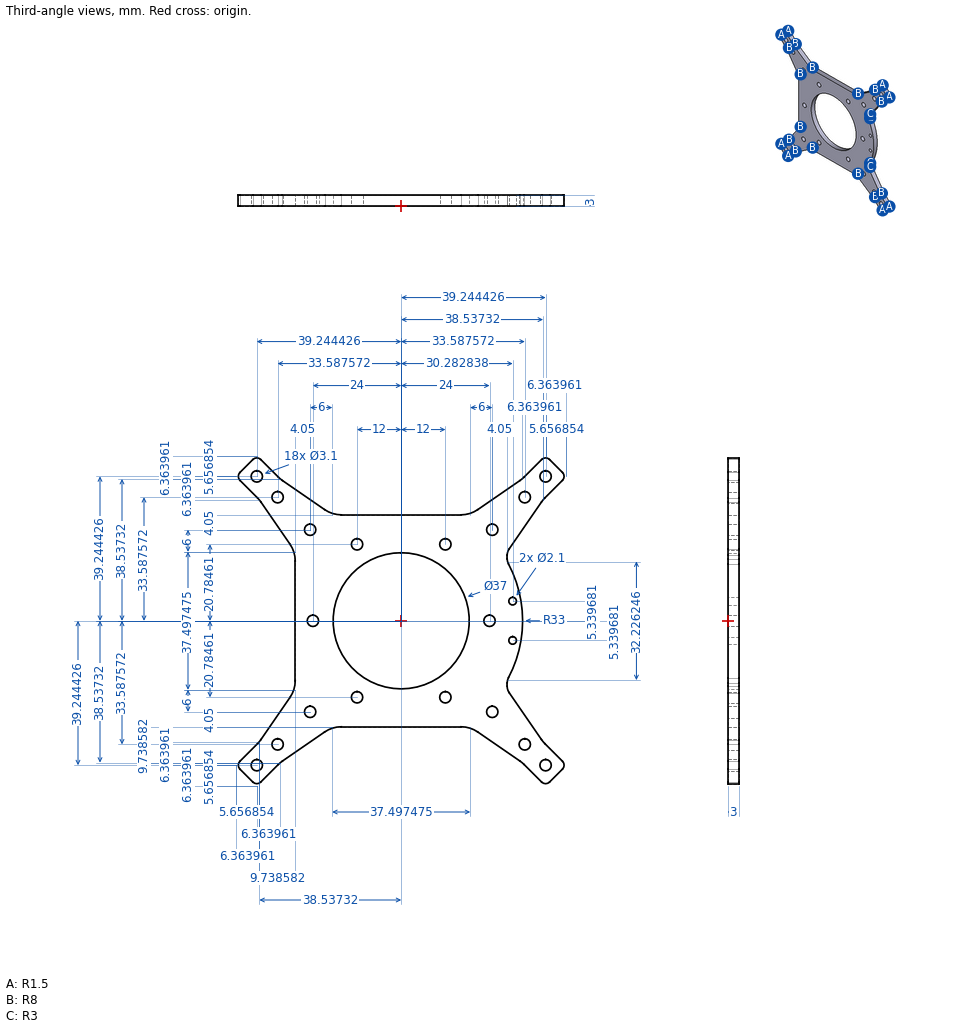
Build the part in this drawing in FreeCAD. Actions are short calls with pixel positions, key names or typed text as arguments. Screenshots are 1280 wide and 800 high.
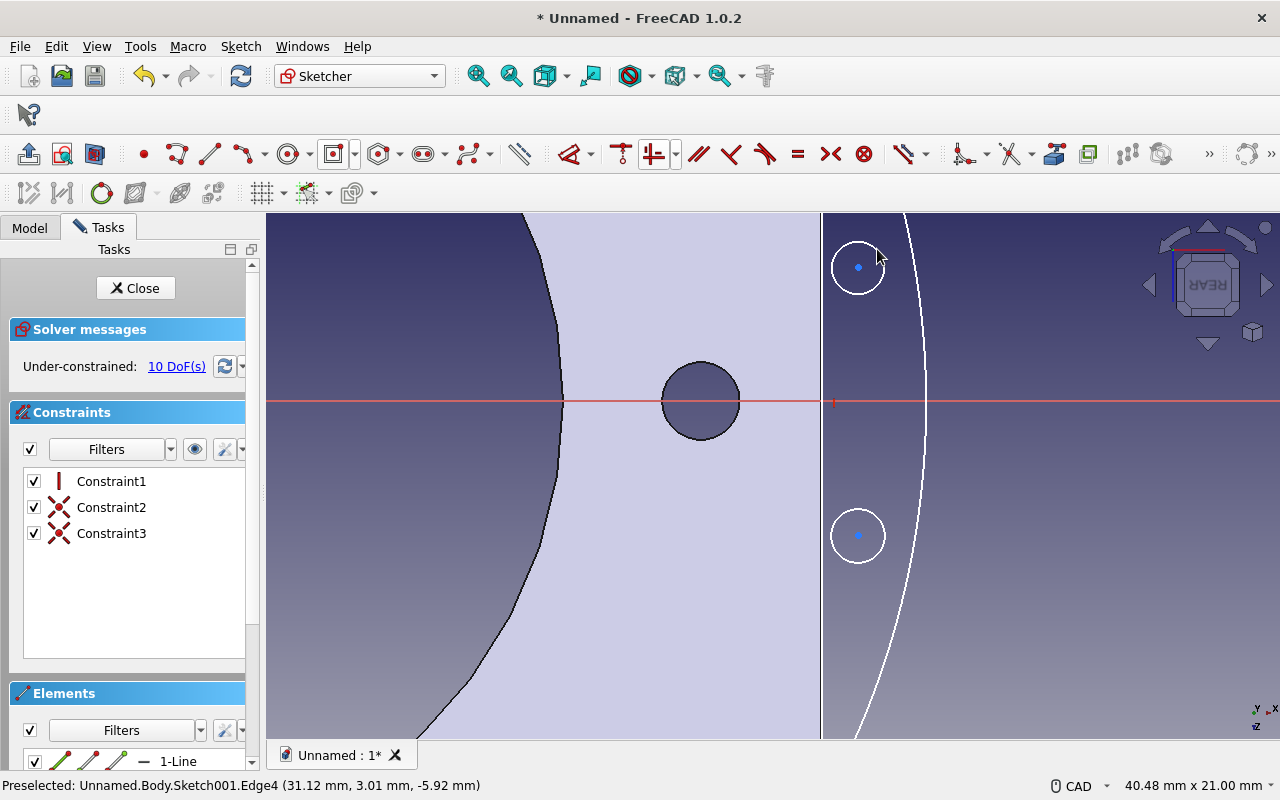
scroll(861, 537, down, 4)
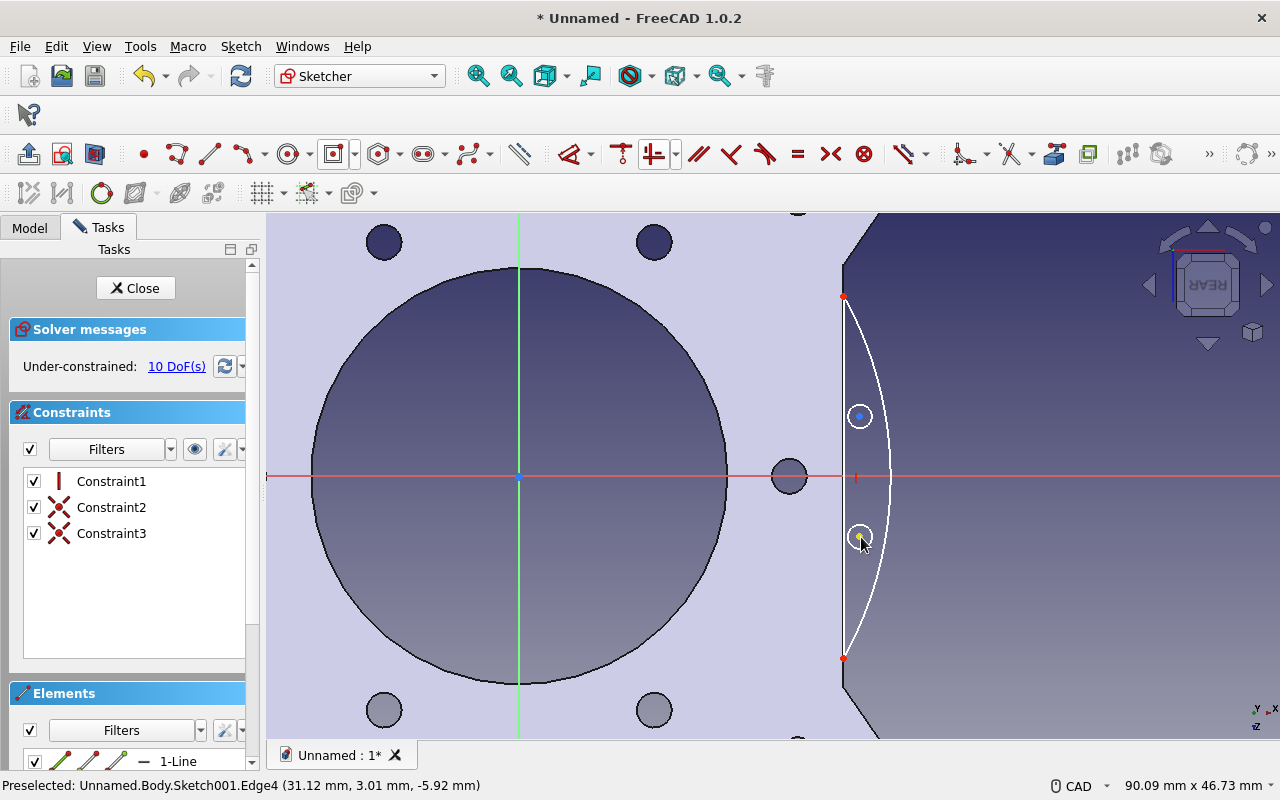
scroll(519, 477, up, 7)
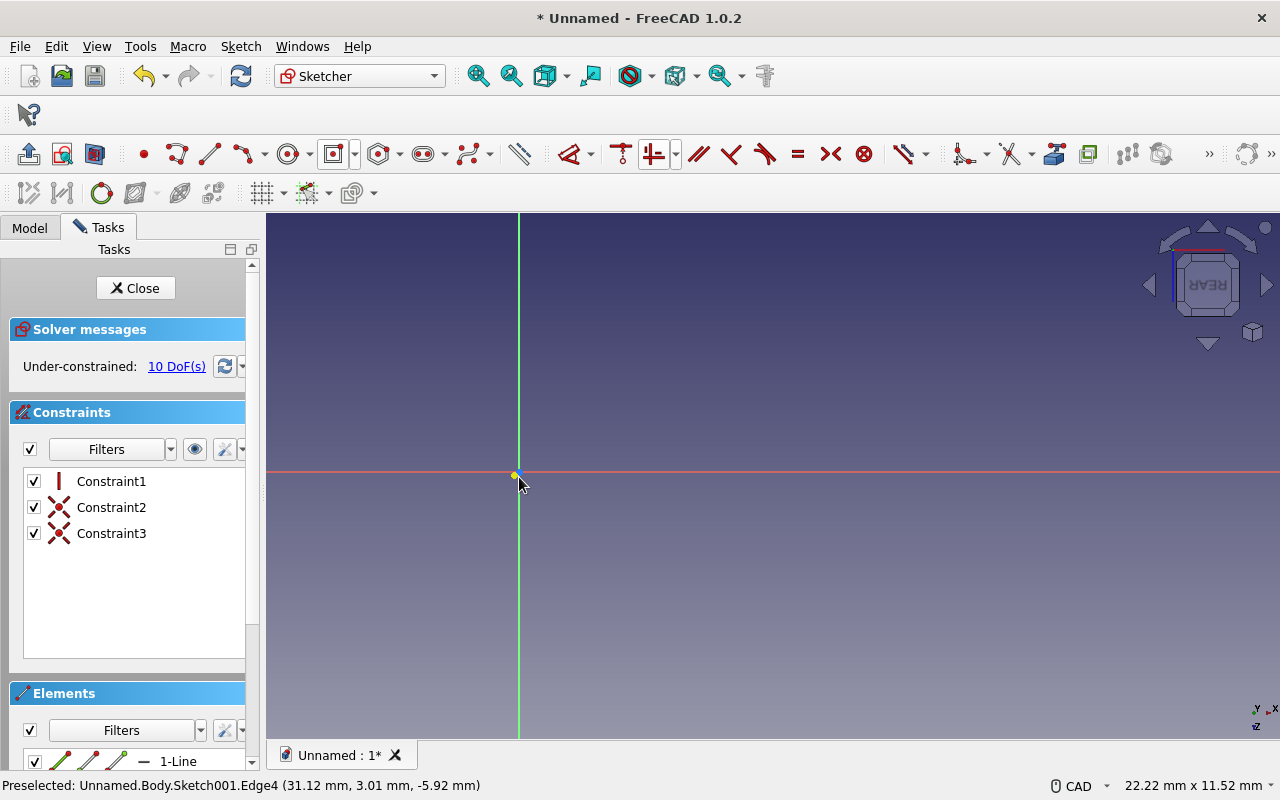
drag(505, 462, 529, 486)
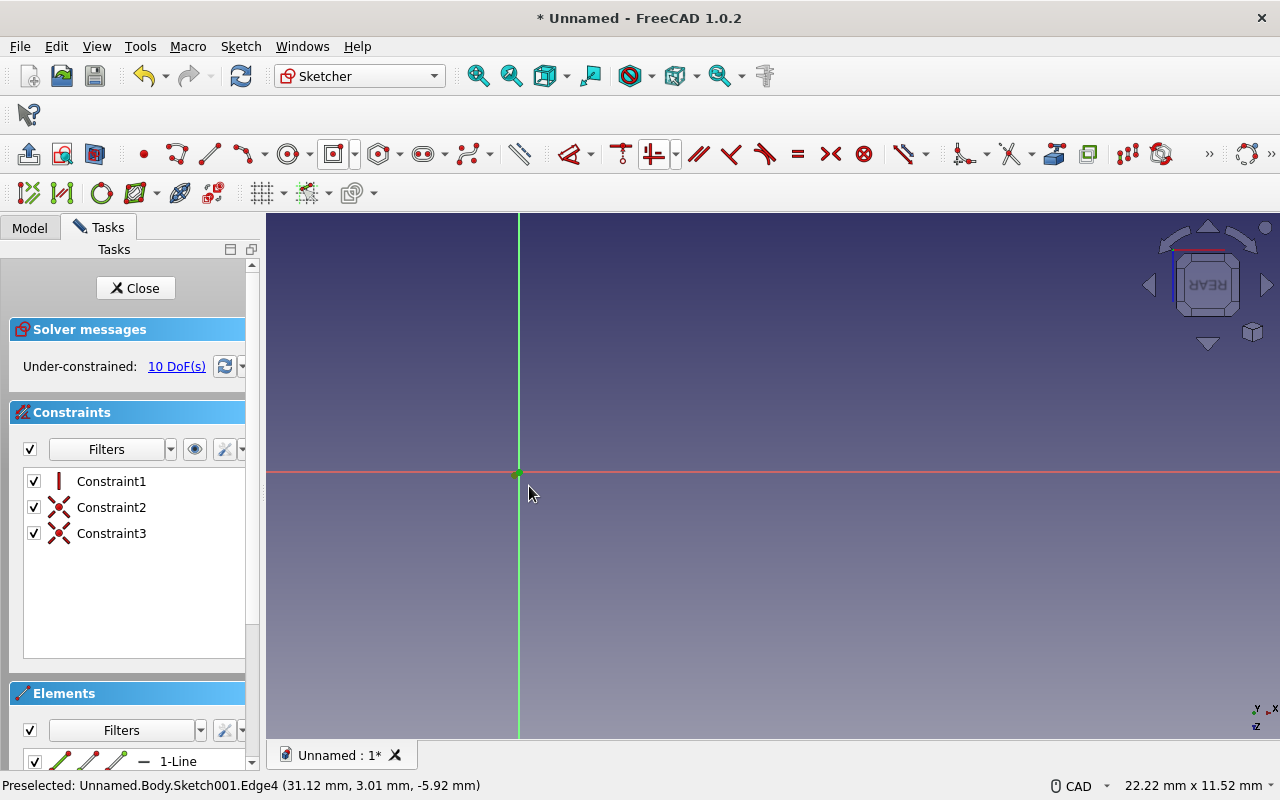
click(621, 154)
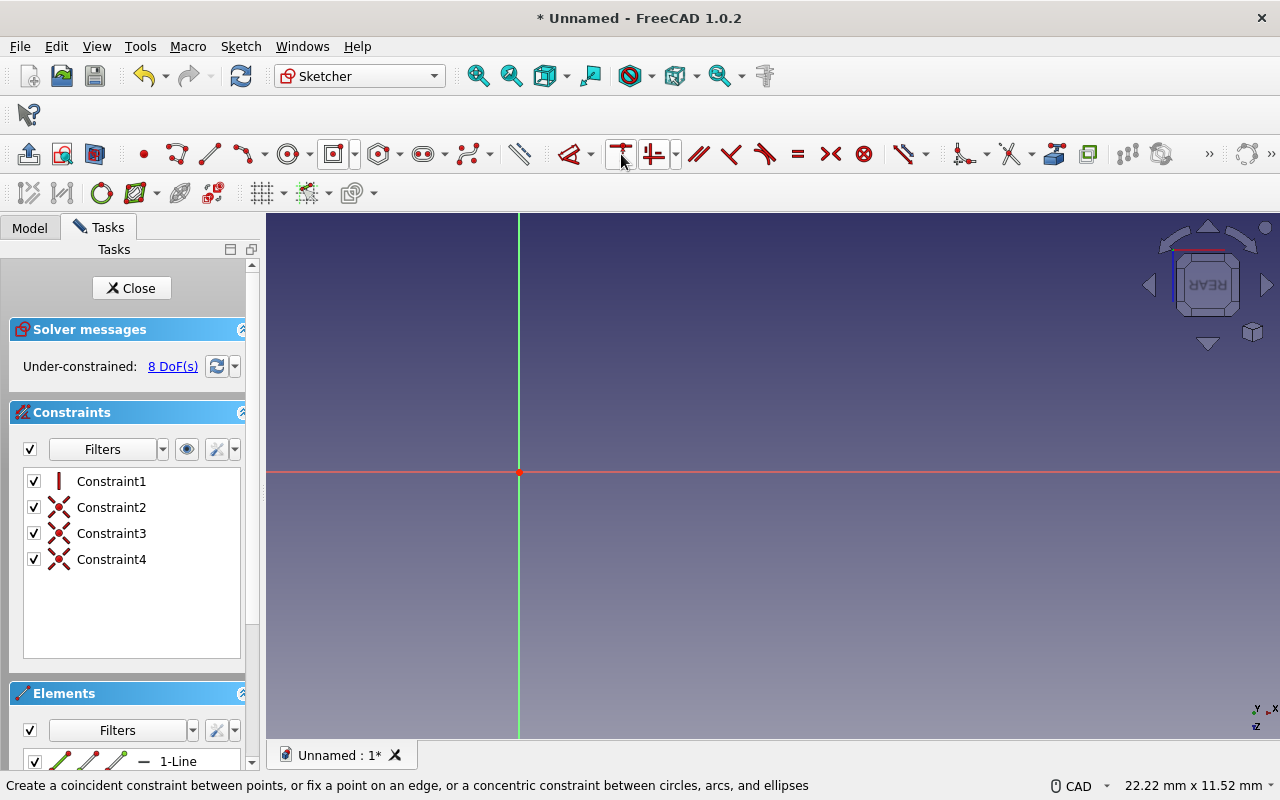
scroll(519, 477, down, 7)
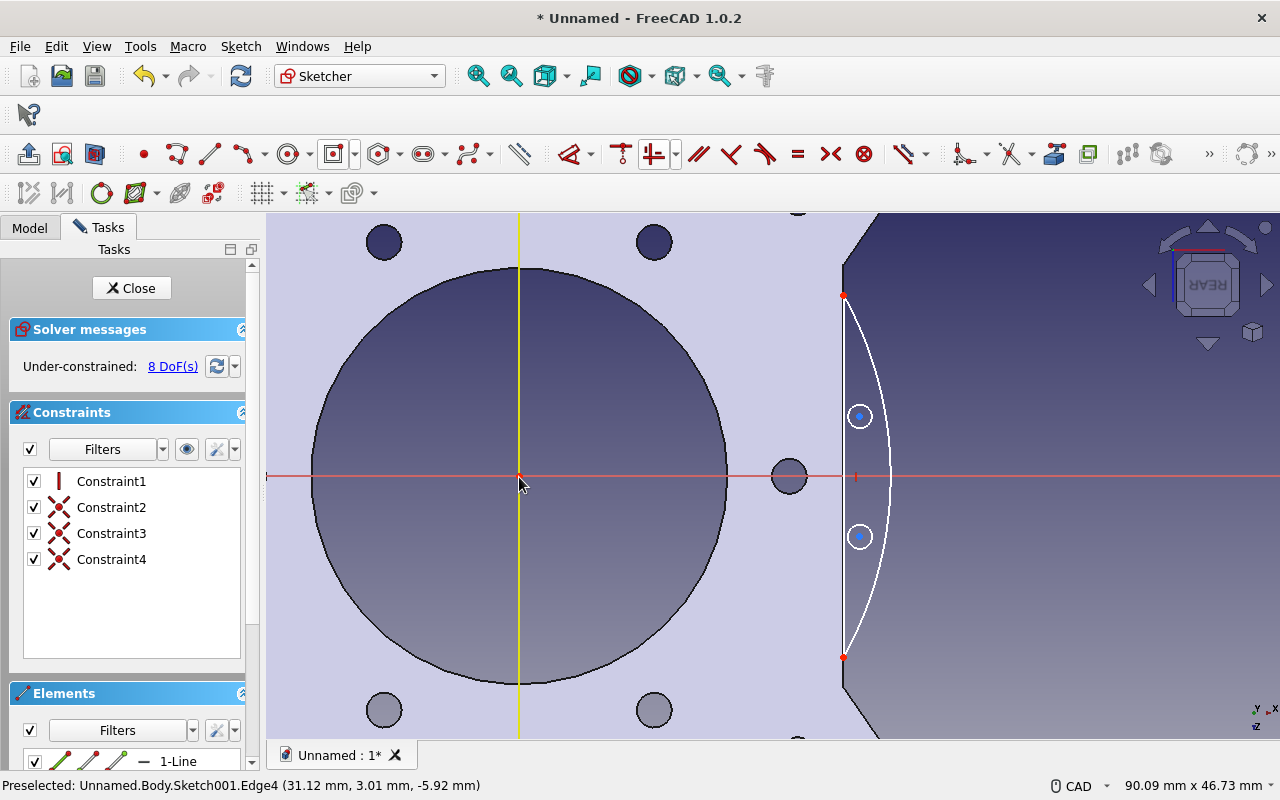
click(868, 528)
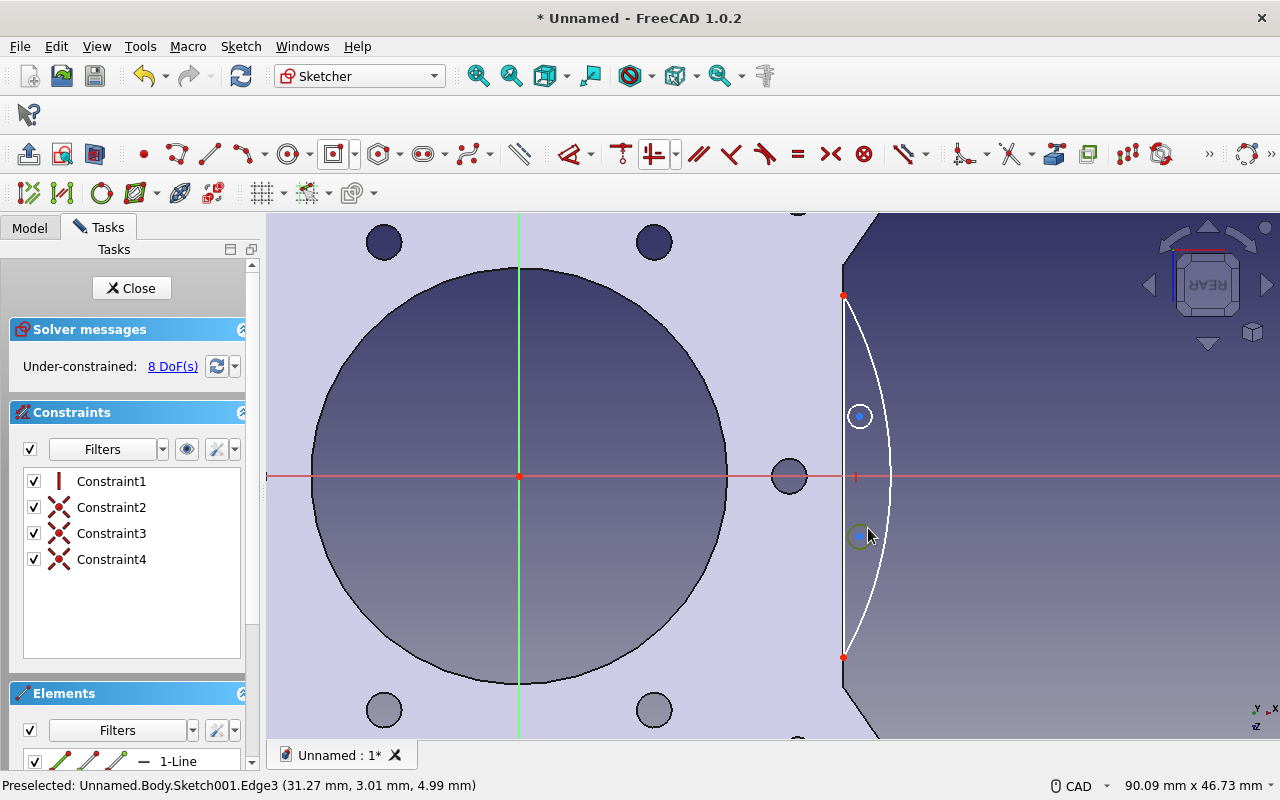
click(868, 408)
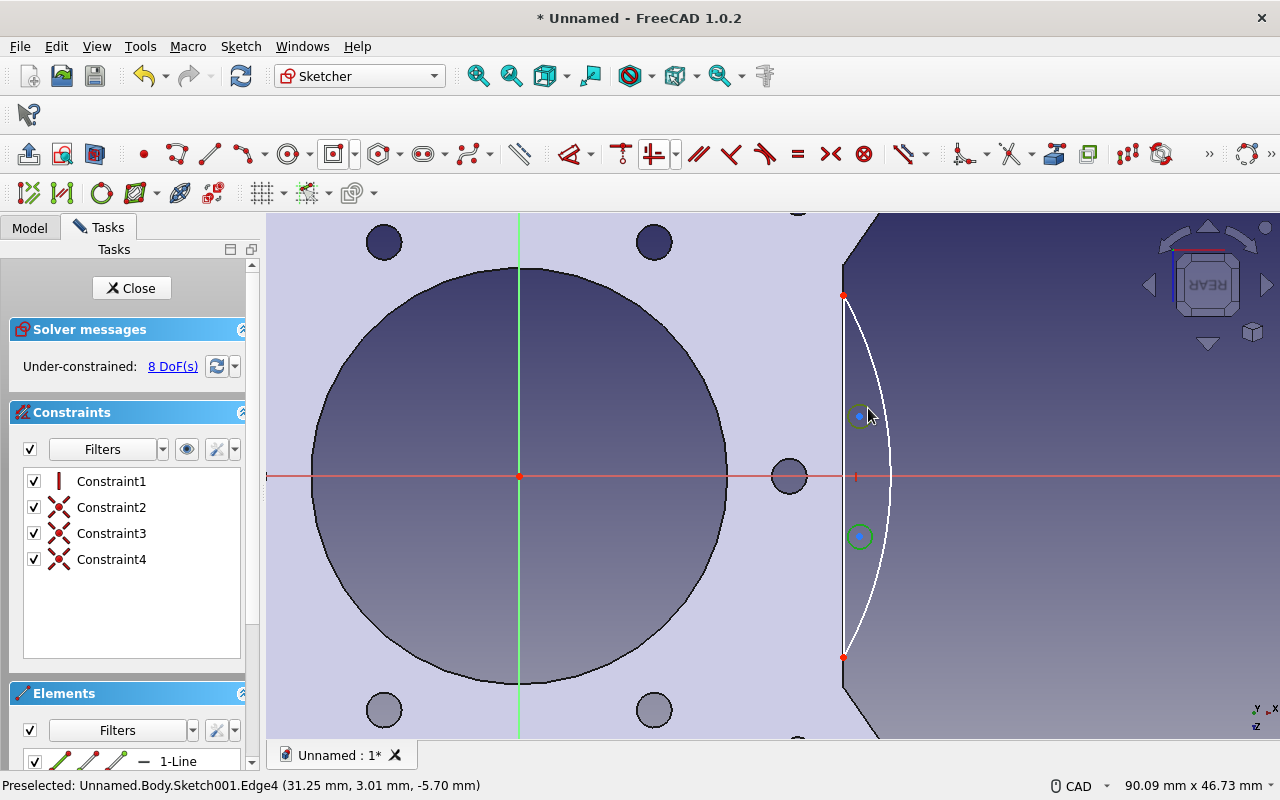
click(798, 154)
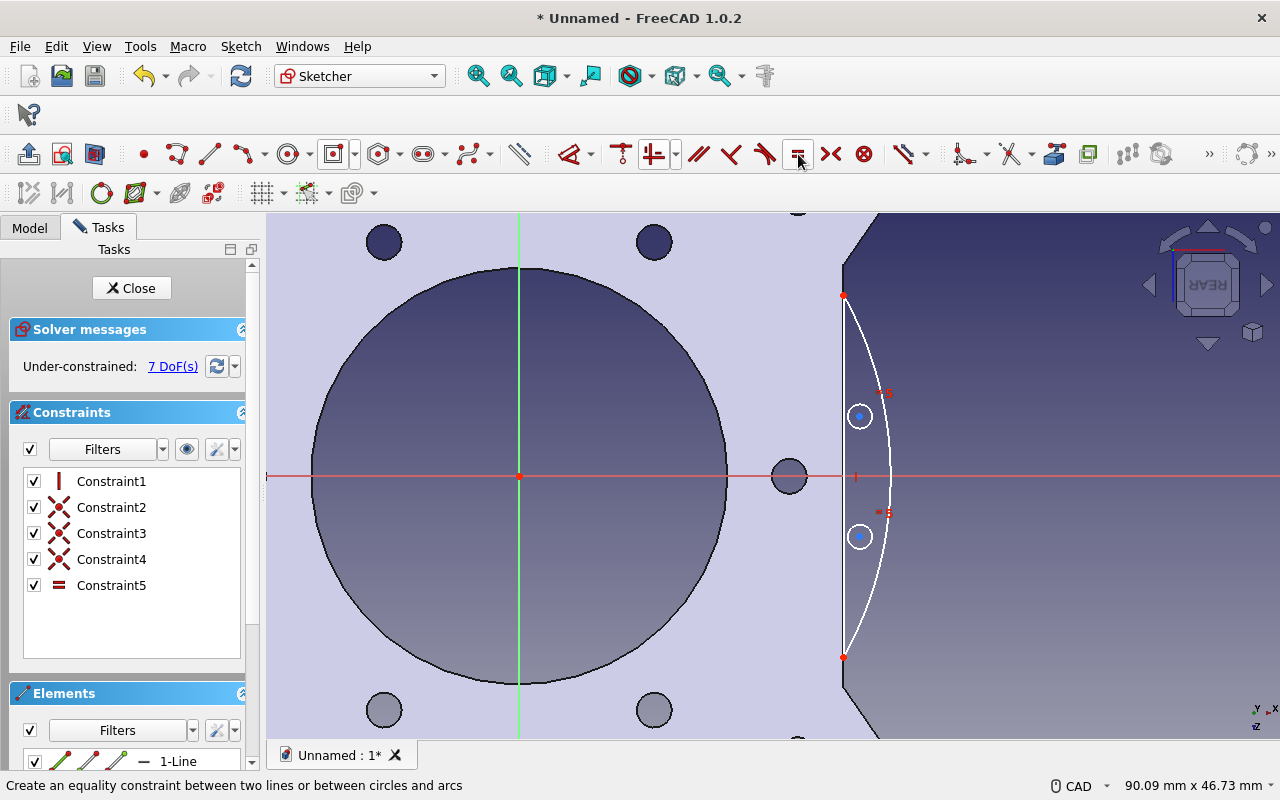
click(860, 537)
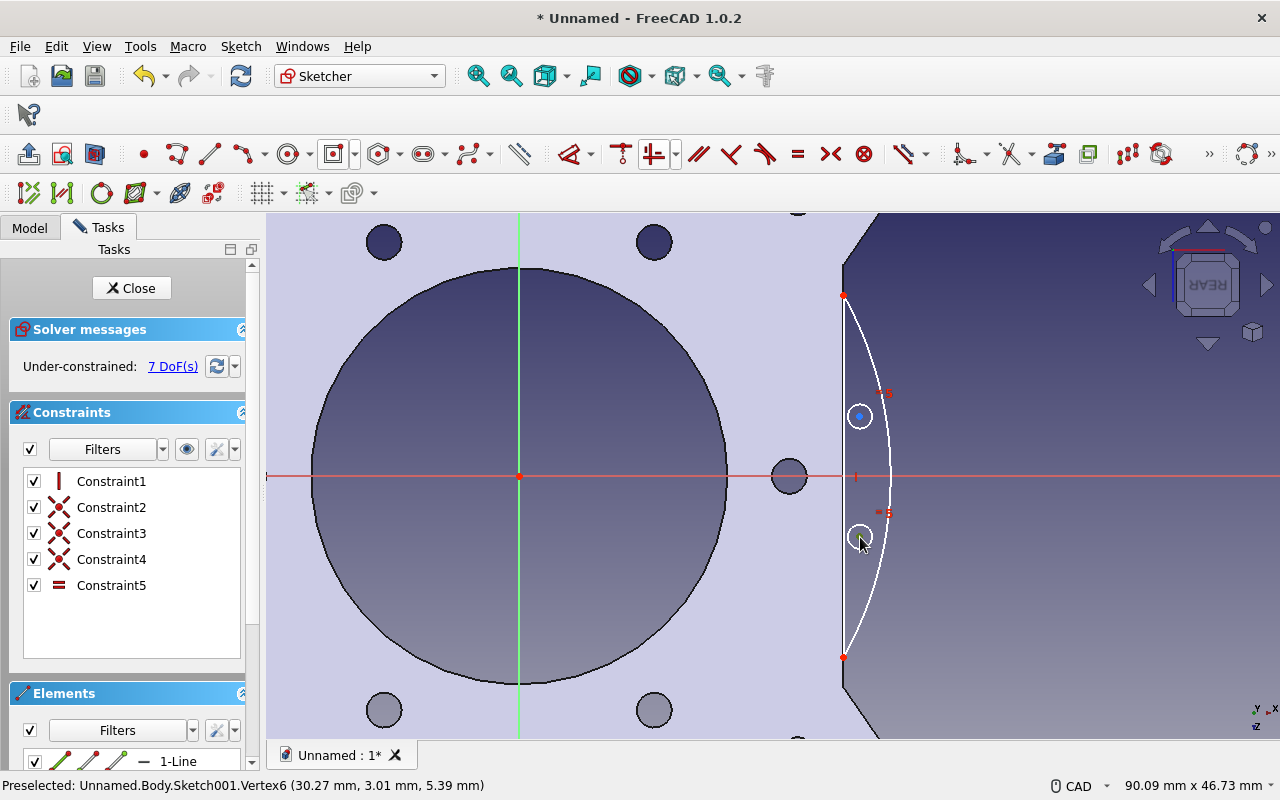
click(860, 416)